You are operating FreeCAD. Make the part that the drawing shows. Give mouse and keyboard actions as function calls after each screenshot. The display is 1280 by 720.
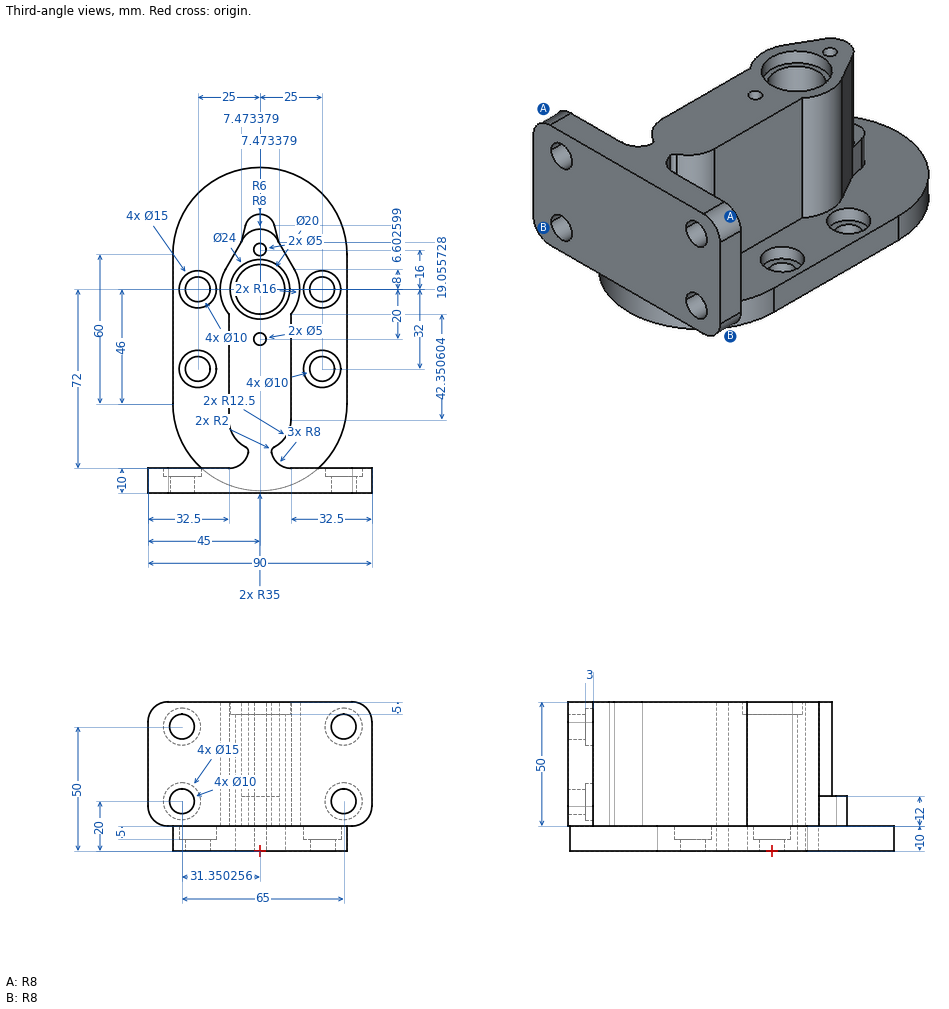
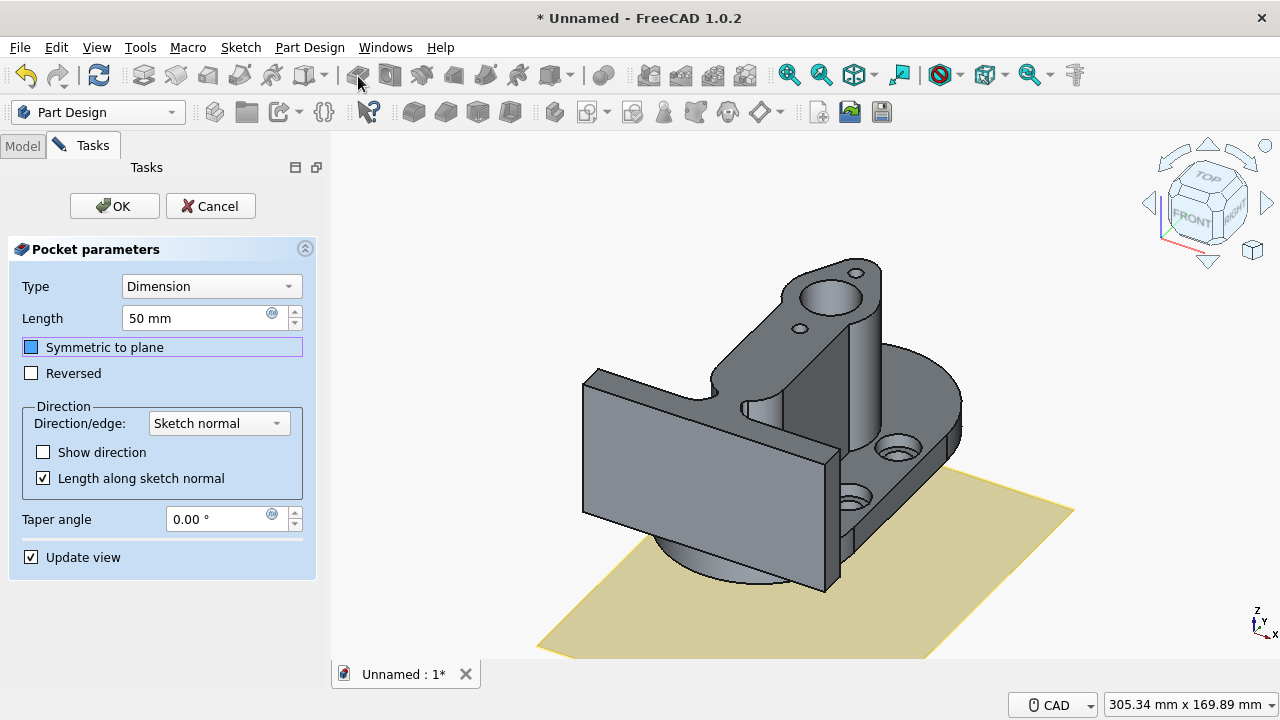
click(30, 373)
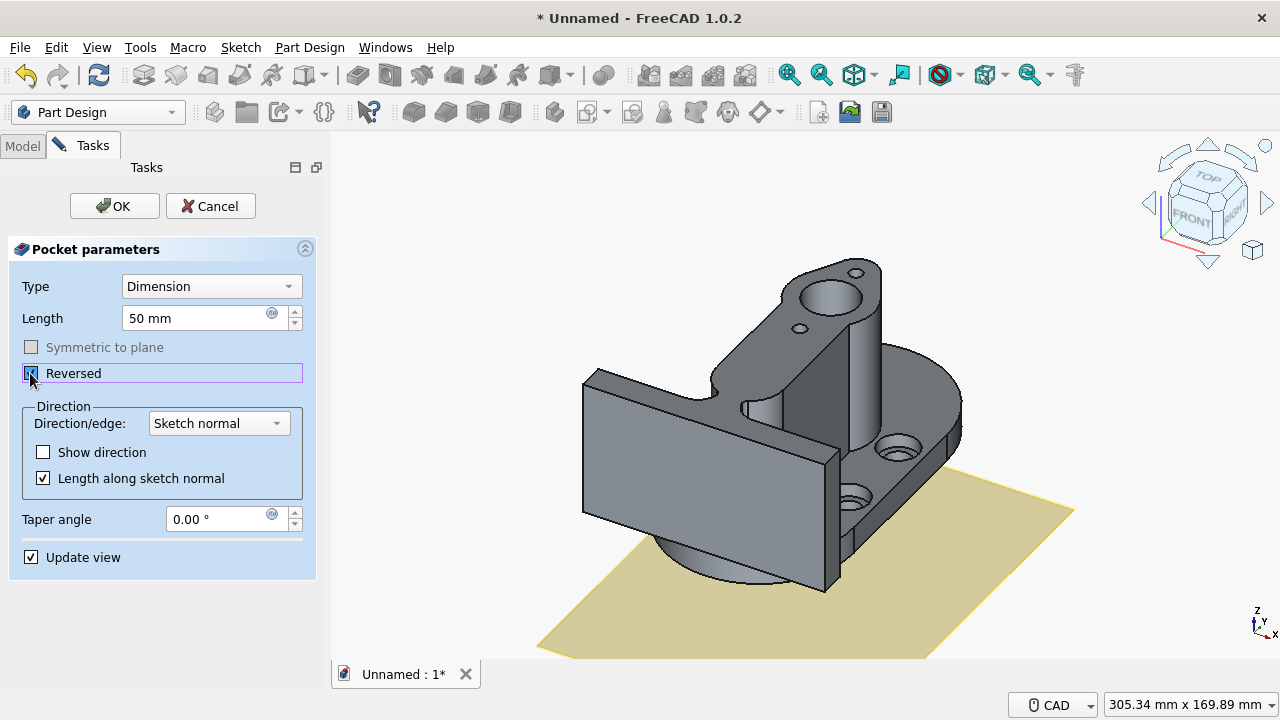
click(115, 206)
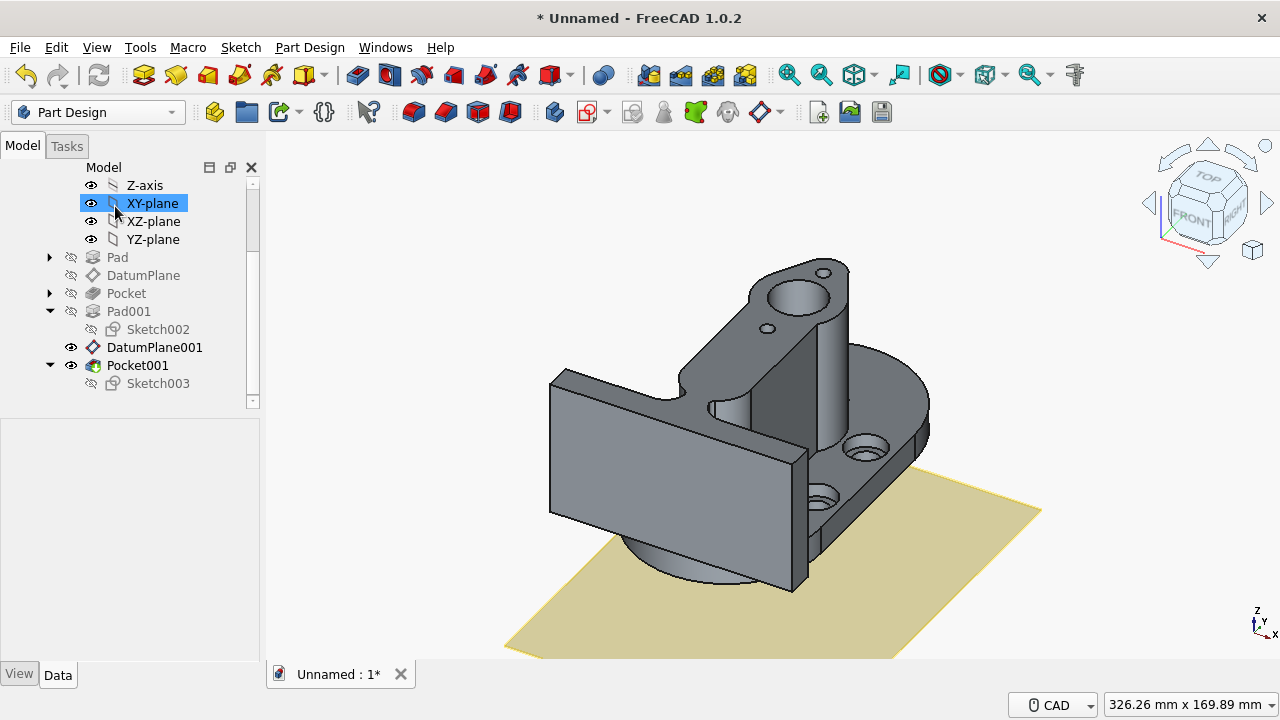
click(116, 347)
key(space)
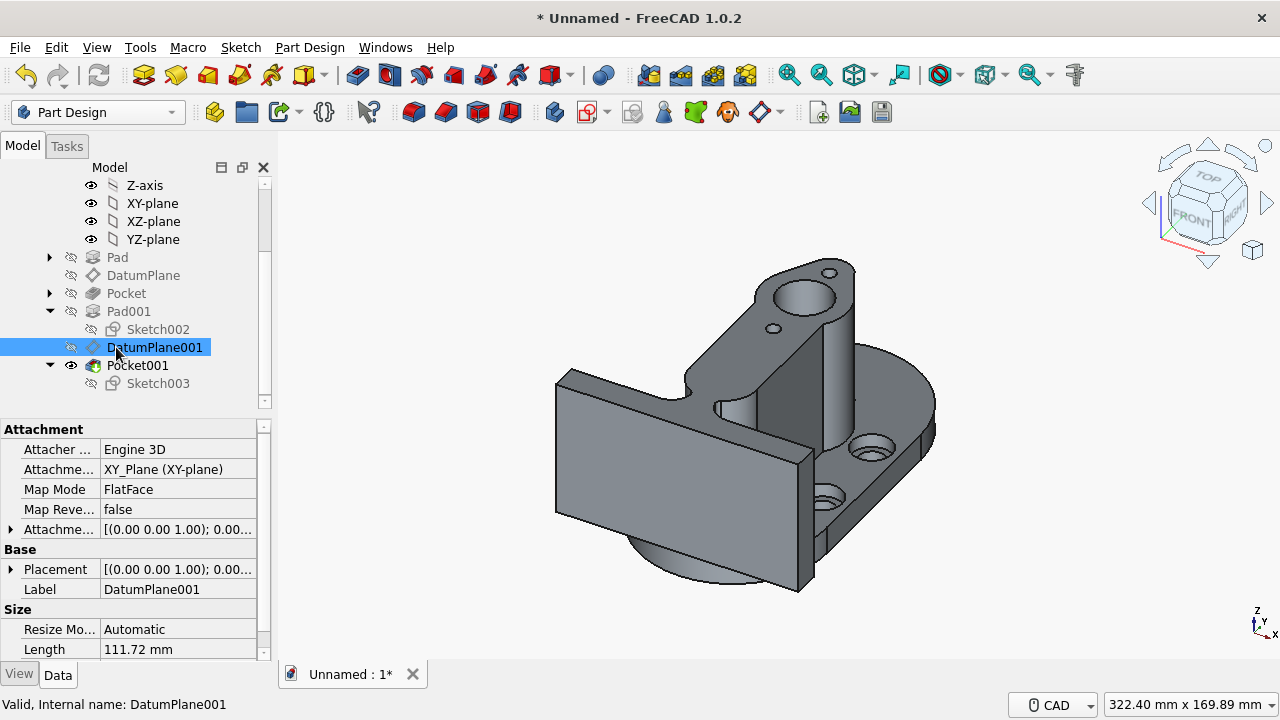
click(736, 365)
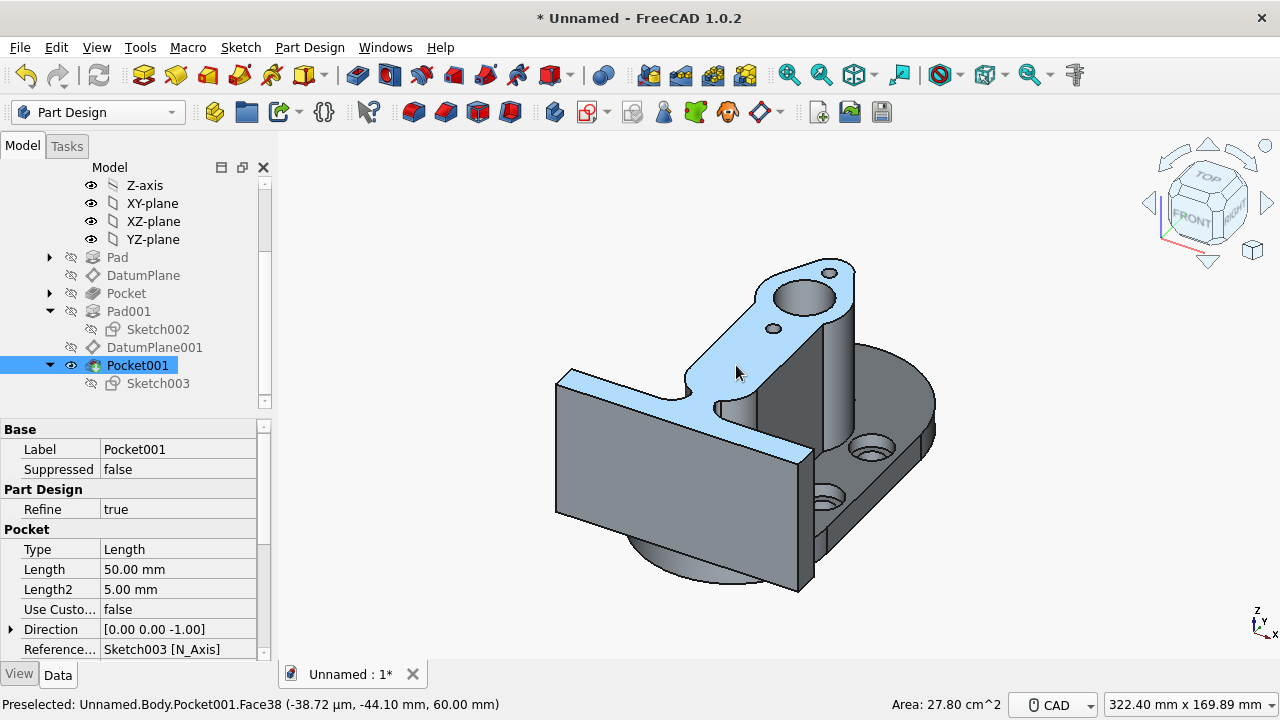
click(588, 112)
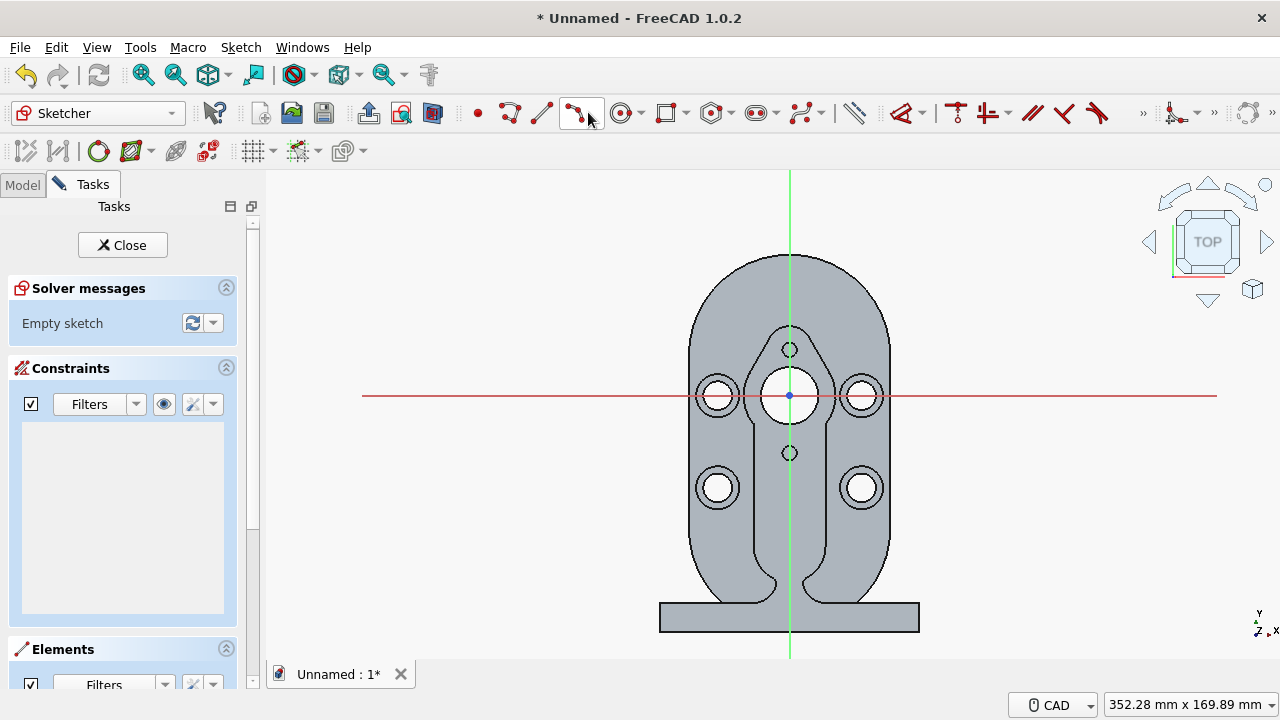
scroll(817, 390, up, 7)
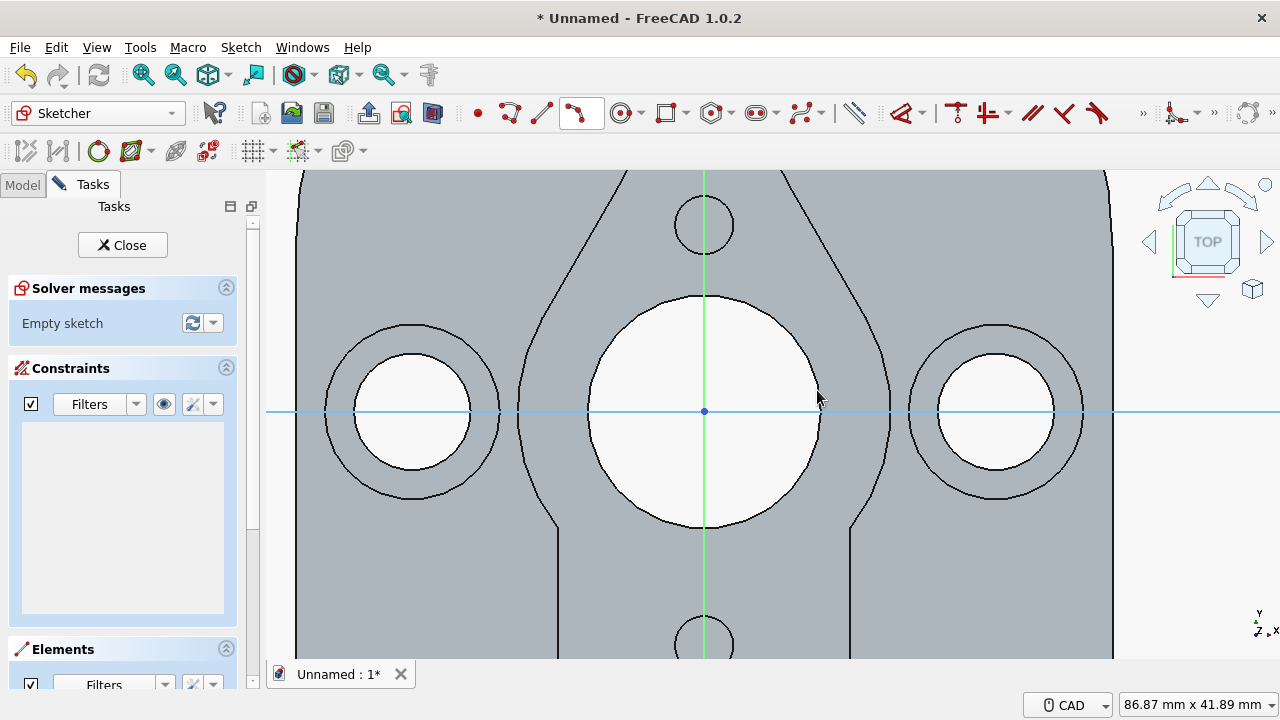
click(622, 114)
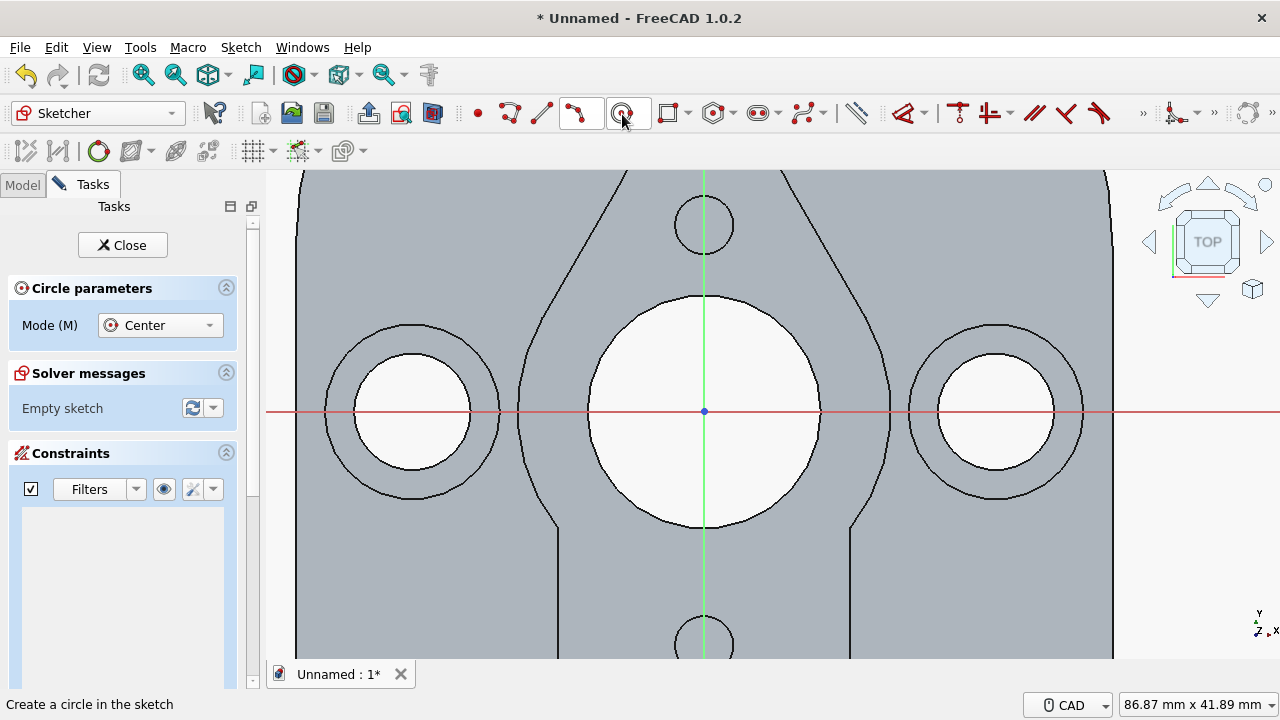
click(704, 412)
click(803, 313)
key(Escape)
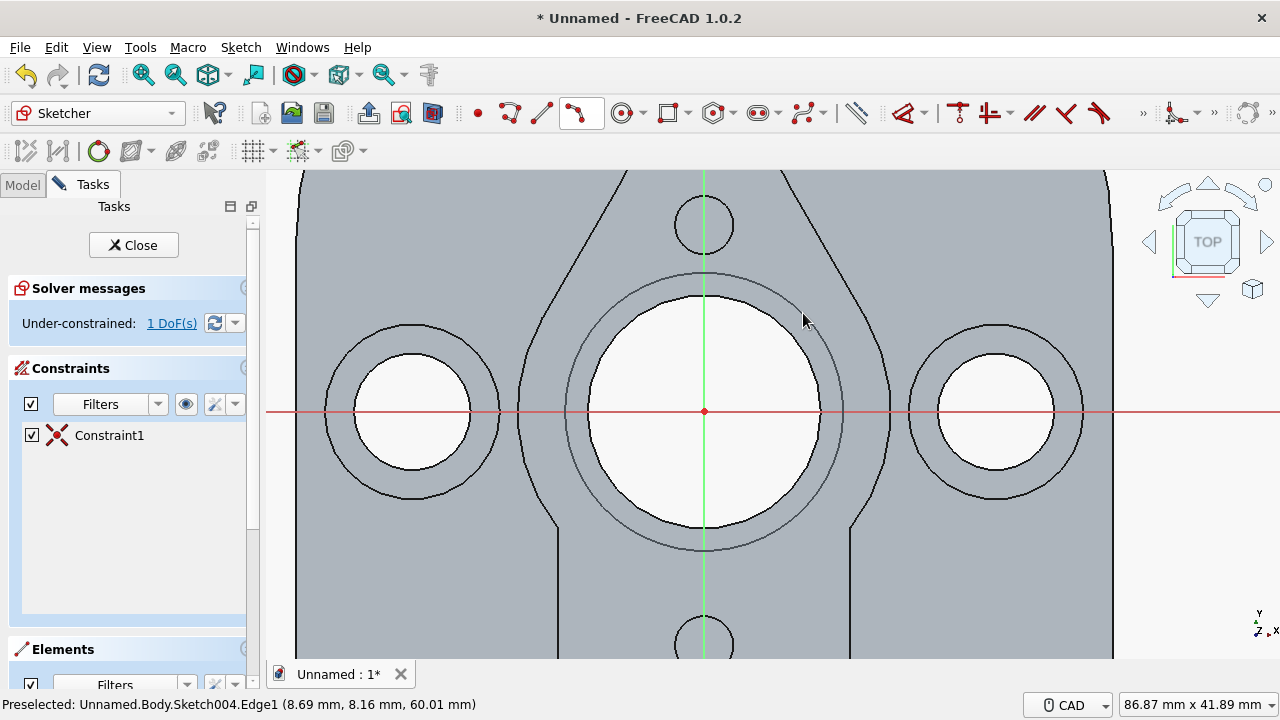
click(904, 114)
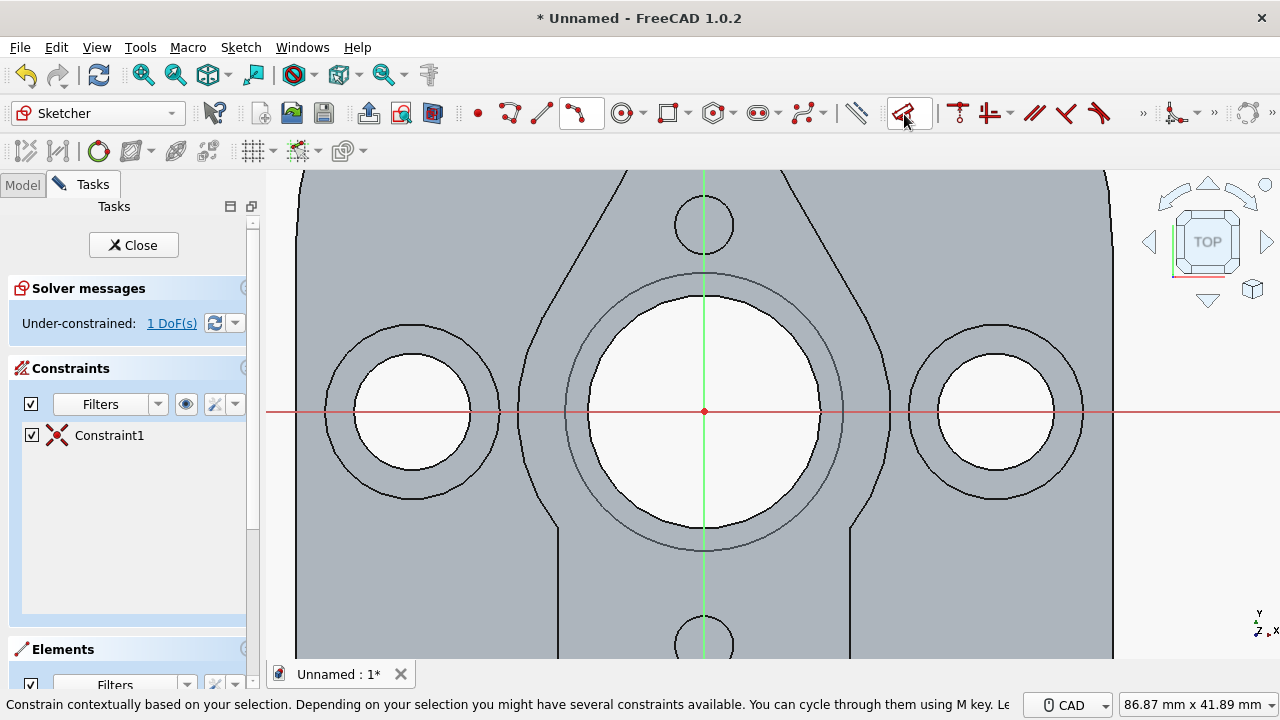
click(802, 313)
click(825, 290)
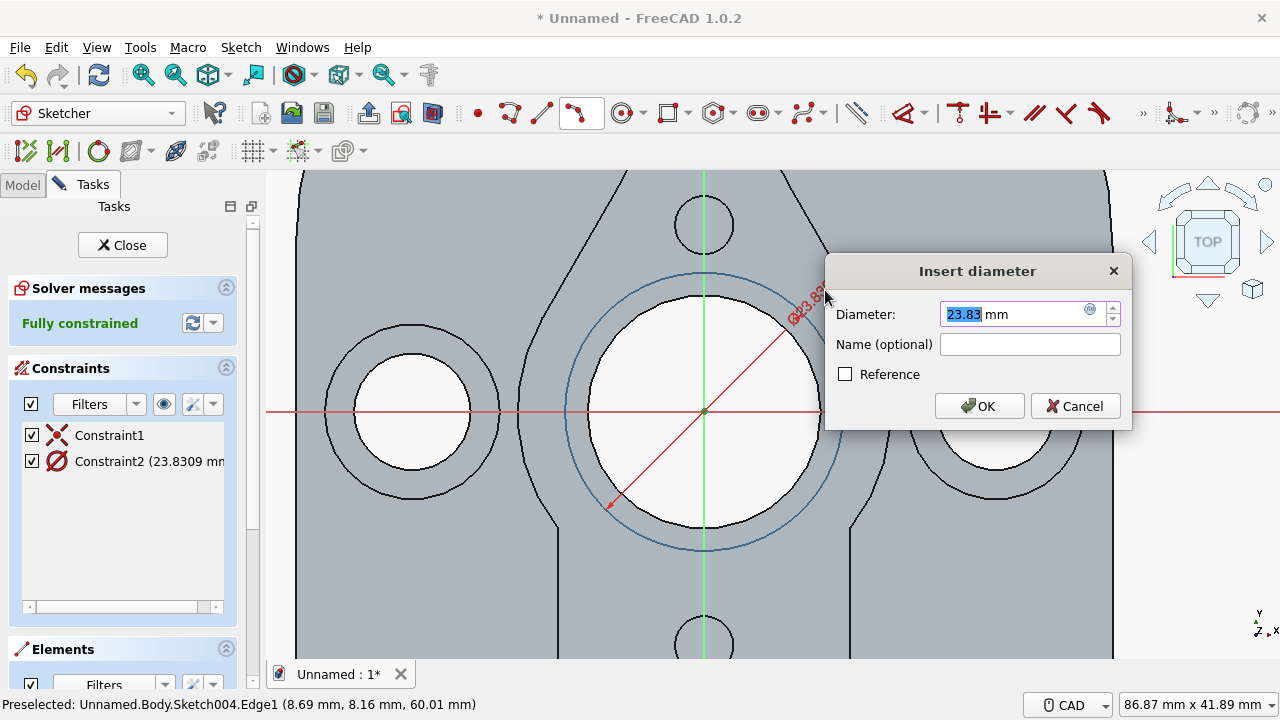
text(24)
key(Return)
key(Escape)